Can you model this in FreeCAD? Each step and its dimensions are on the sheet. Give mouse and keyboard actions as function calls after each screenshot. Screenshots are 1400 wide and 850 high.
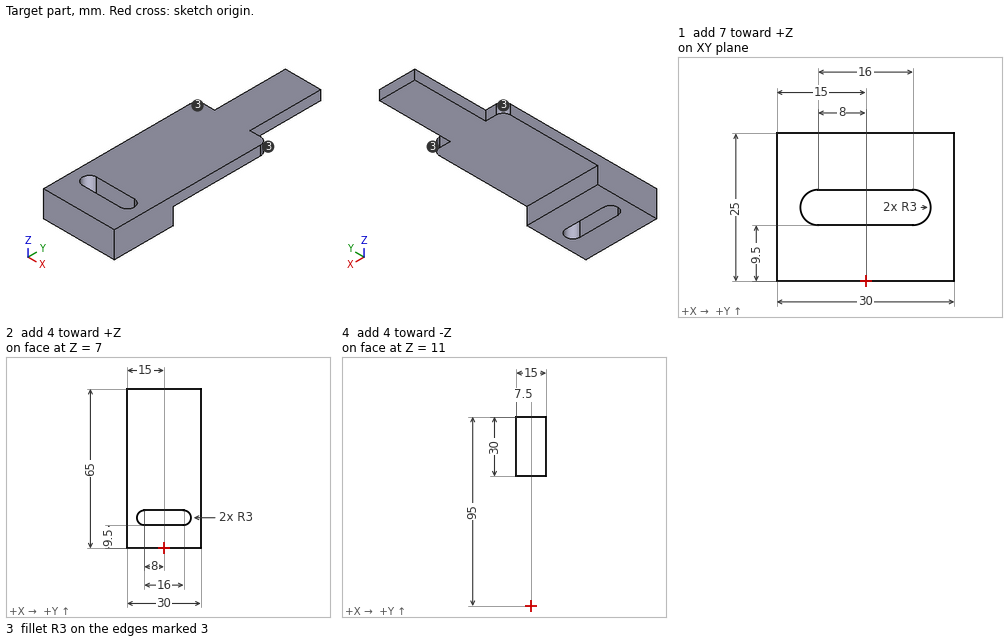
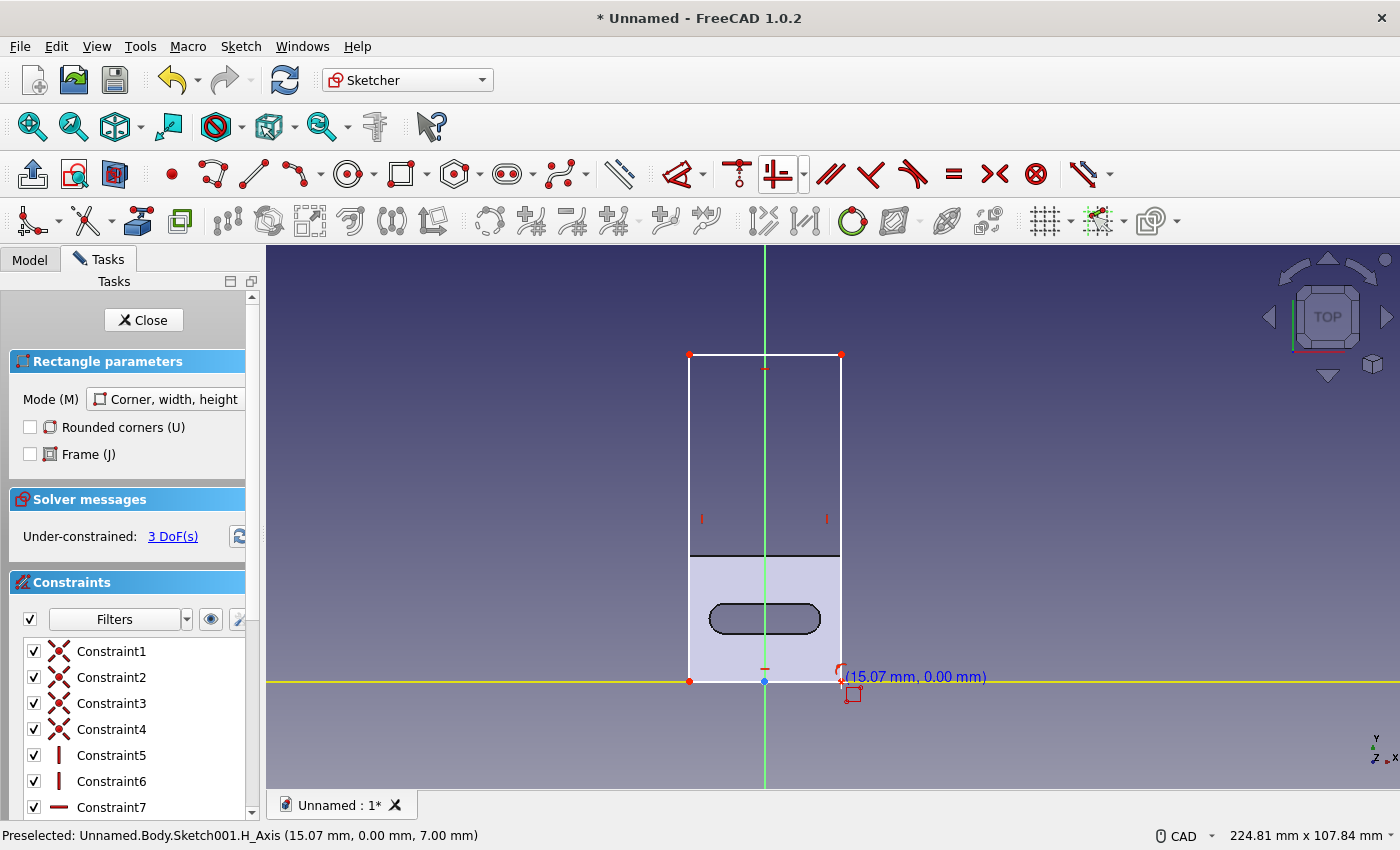
click(506, 174)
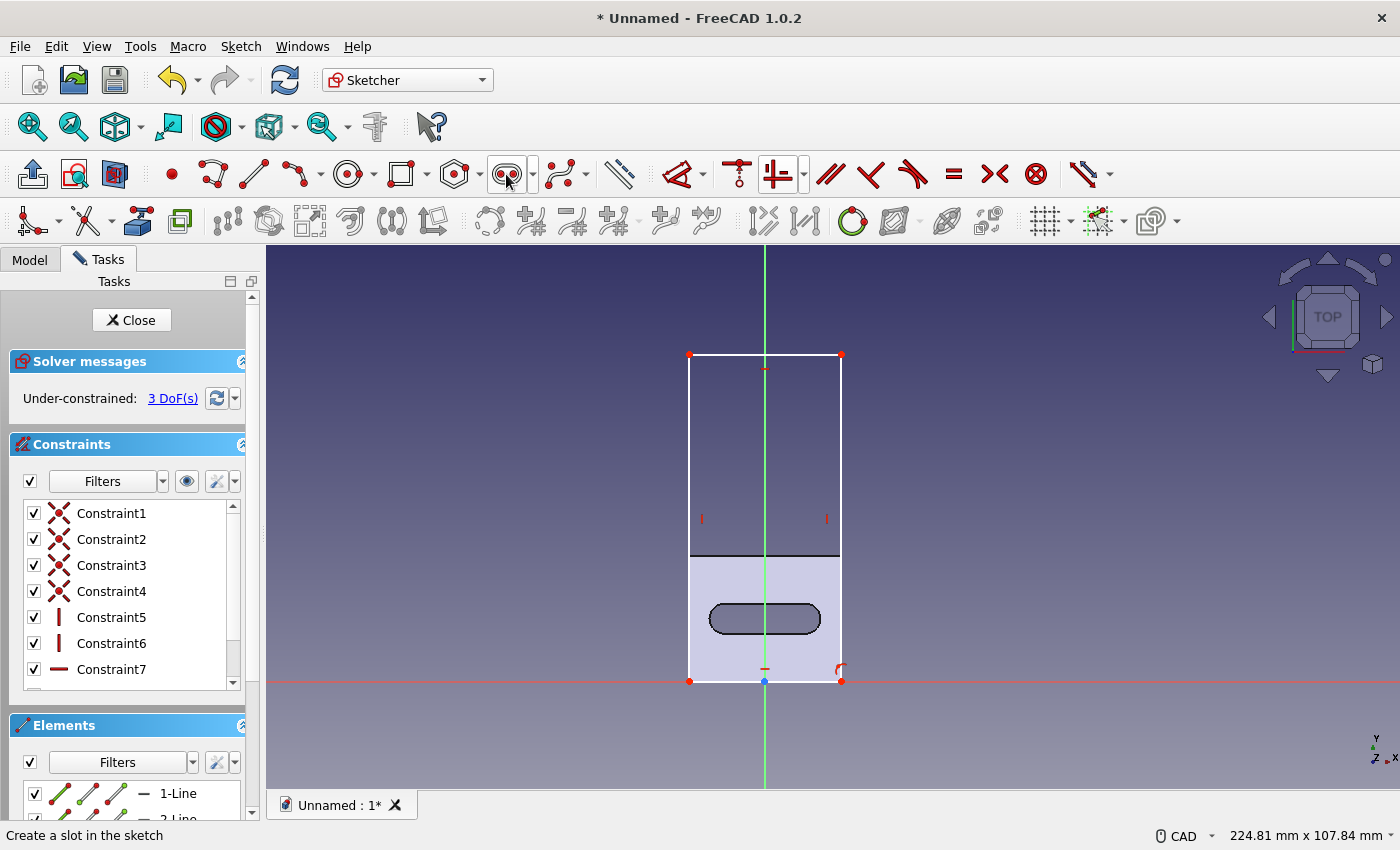
scroll(725, 619, up, 3)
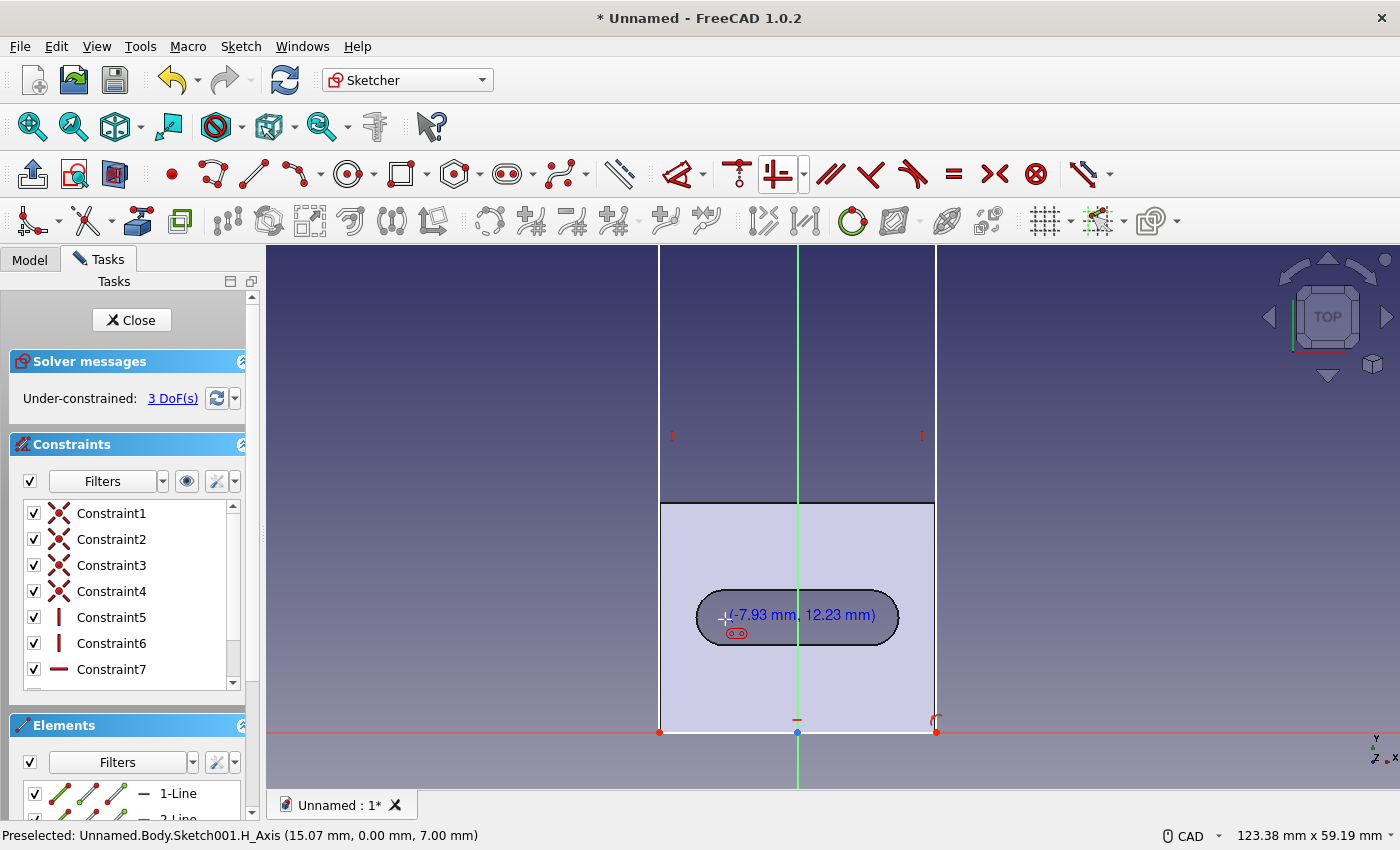
click(724, 618)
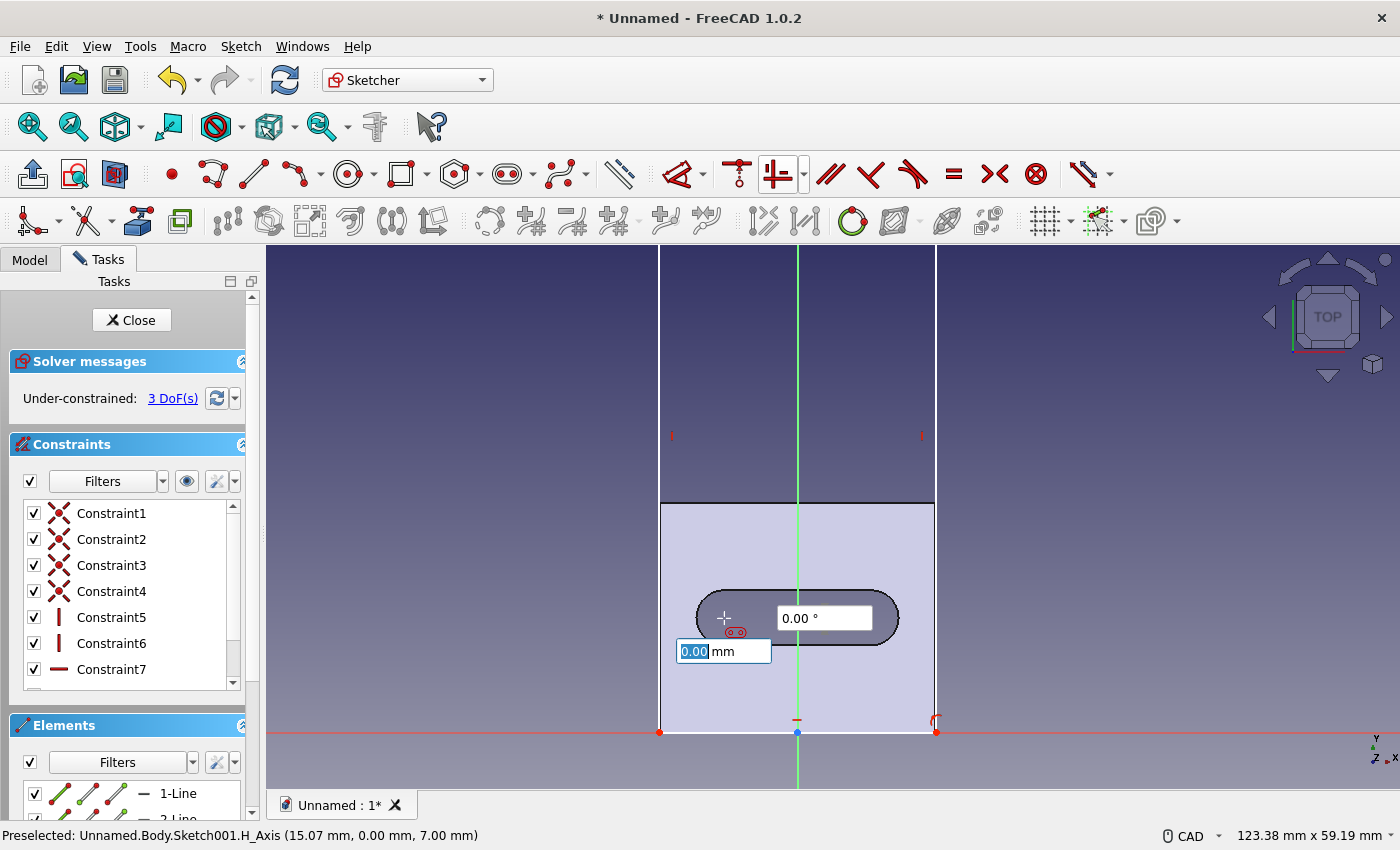
click(871, 618)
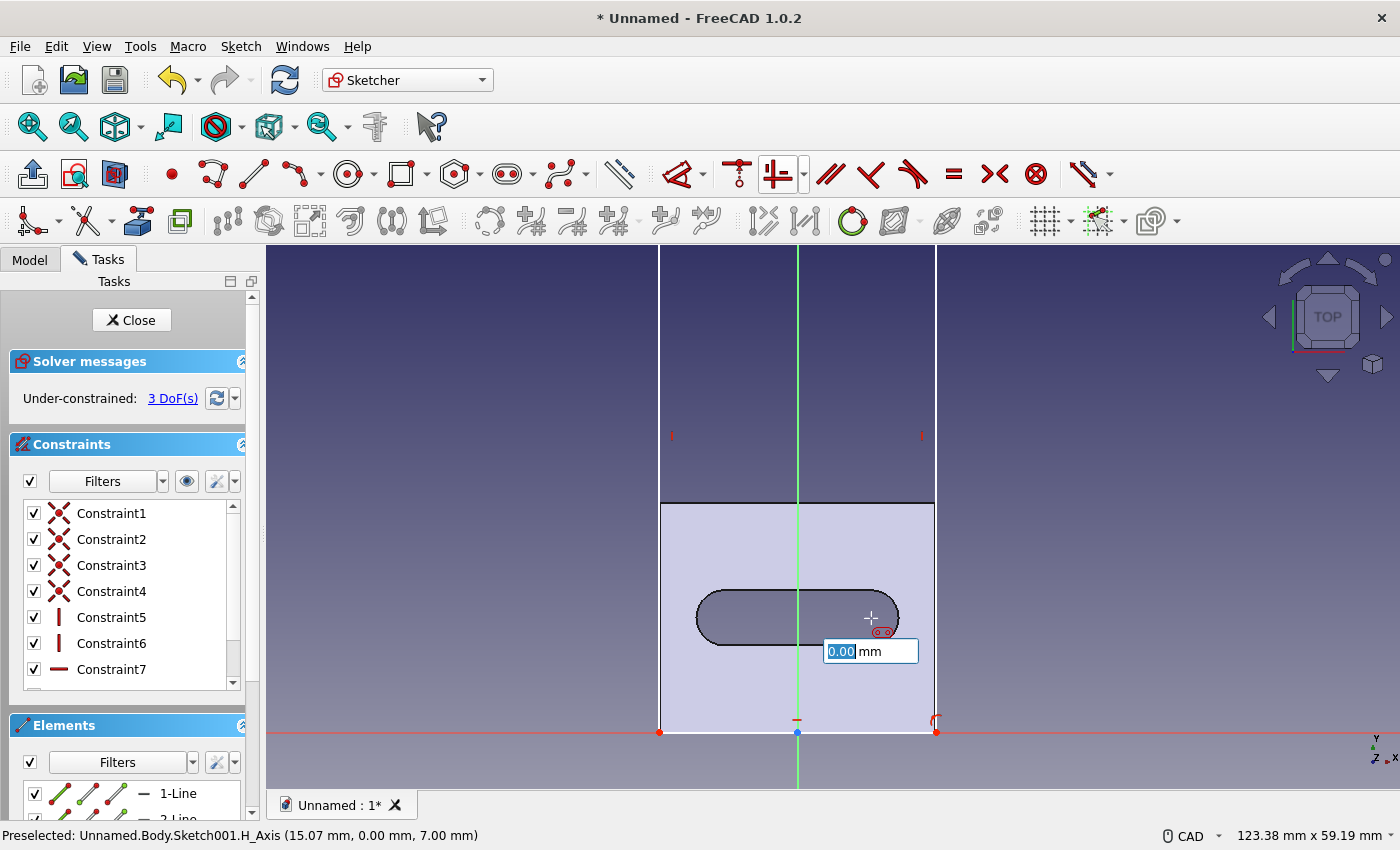
click(820, 645)
key(Escape)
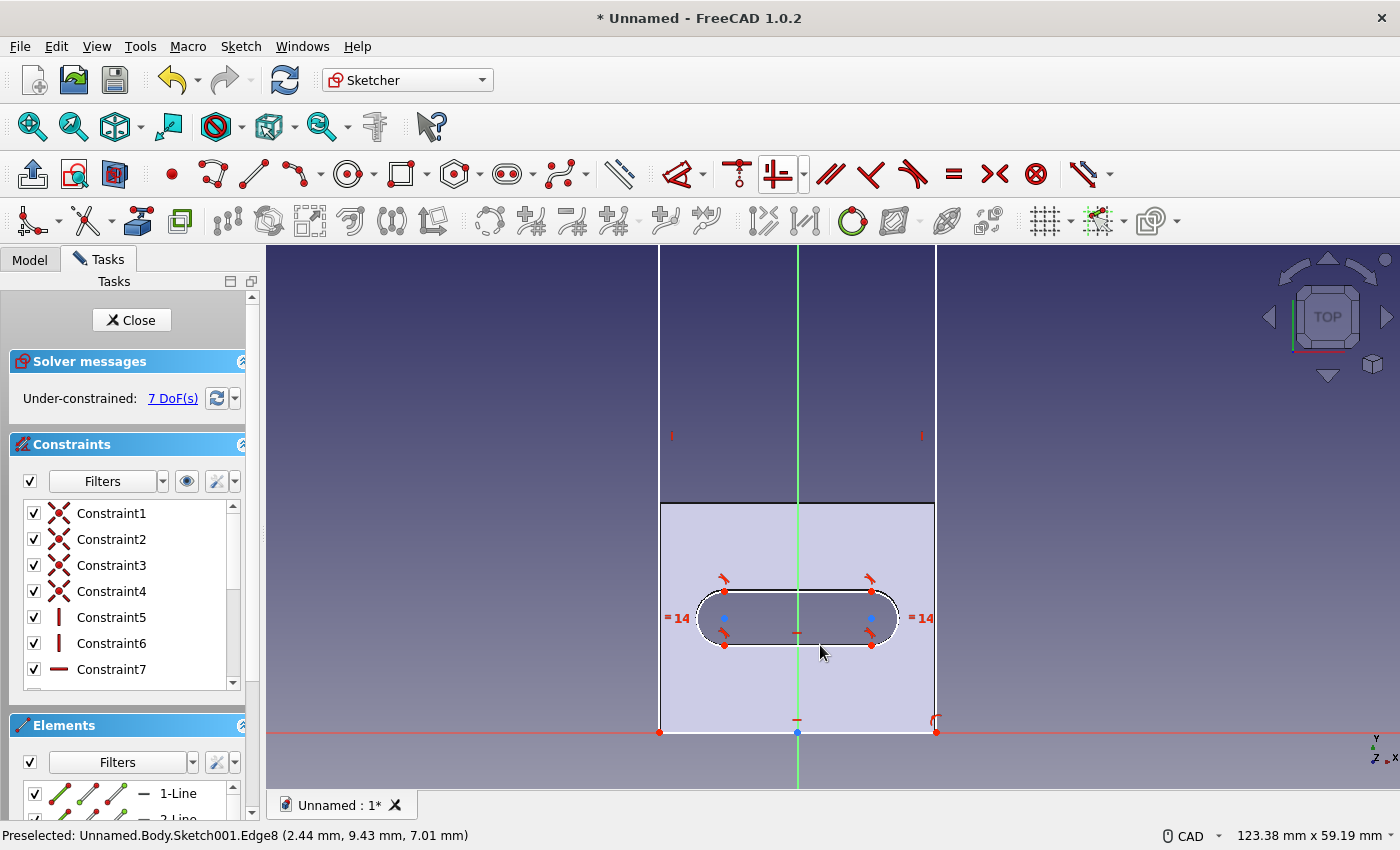
click(676, 174)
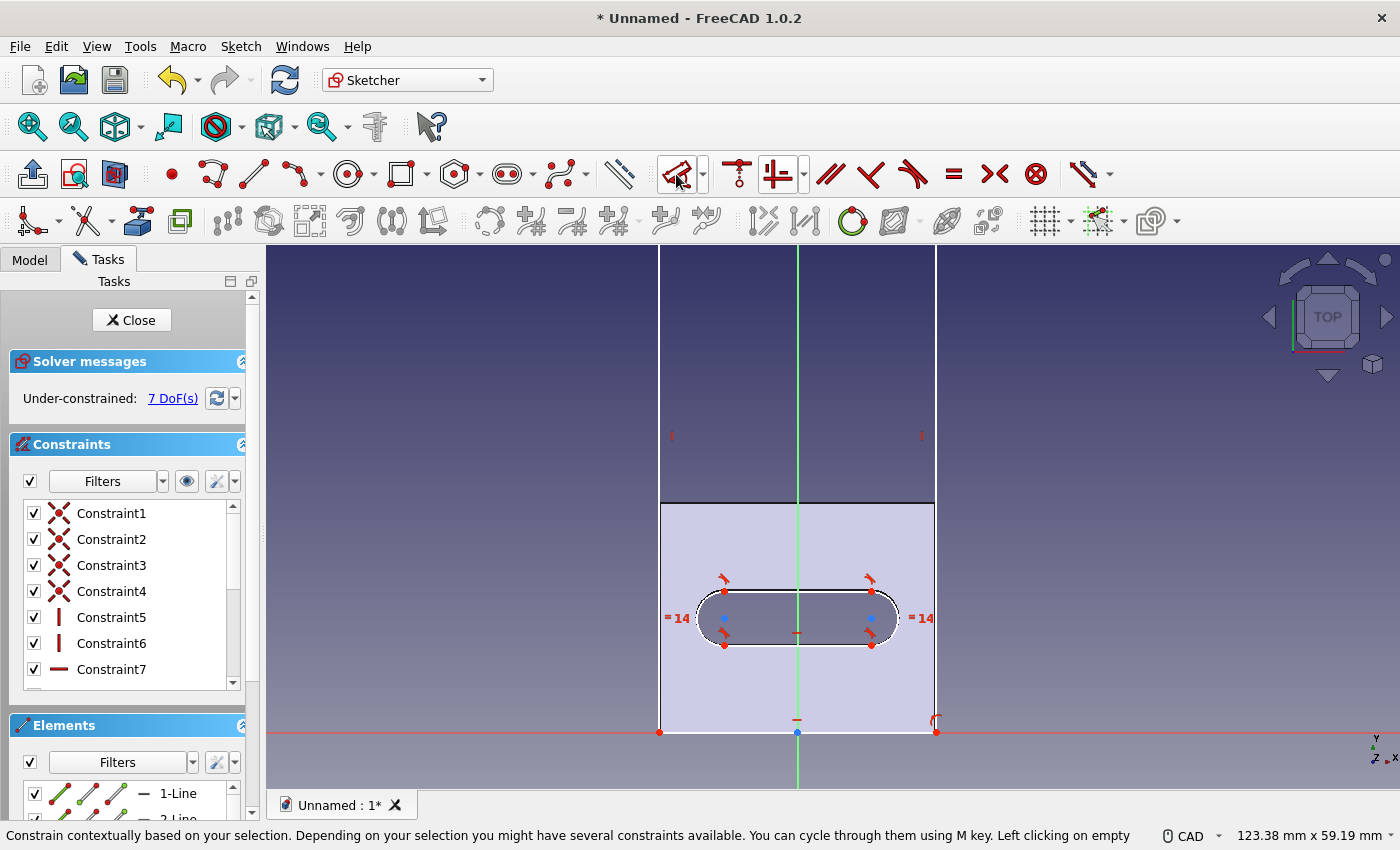
scroll(702, 603, up, 2)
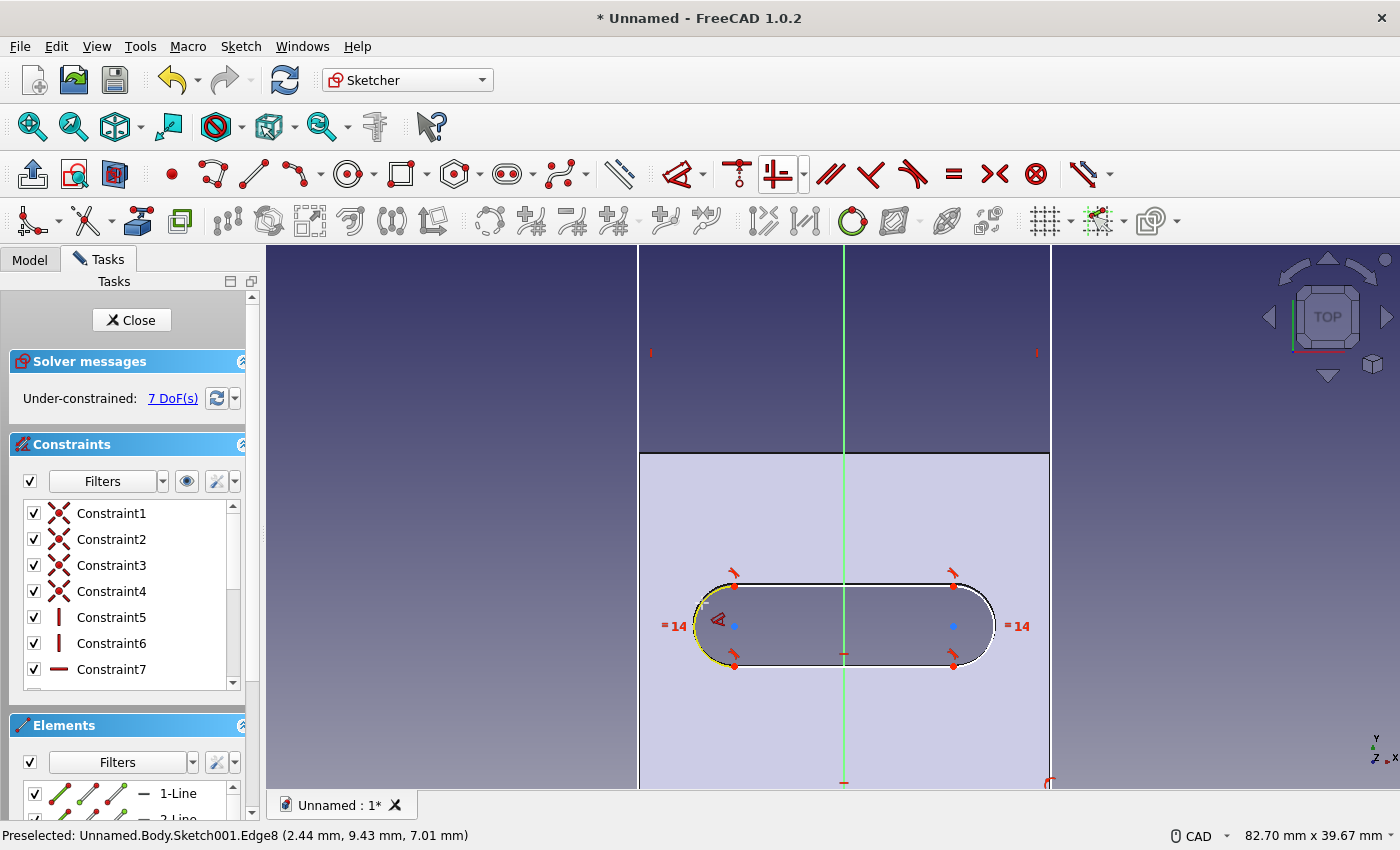
click(702, 603)
click(676, 584)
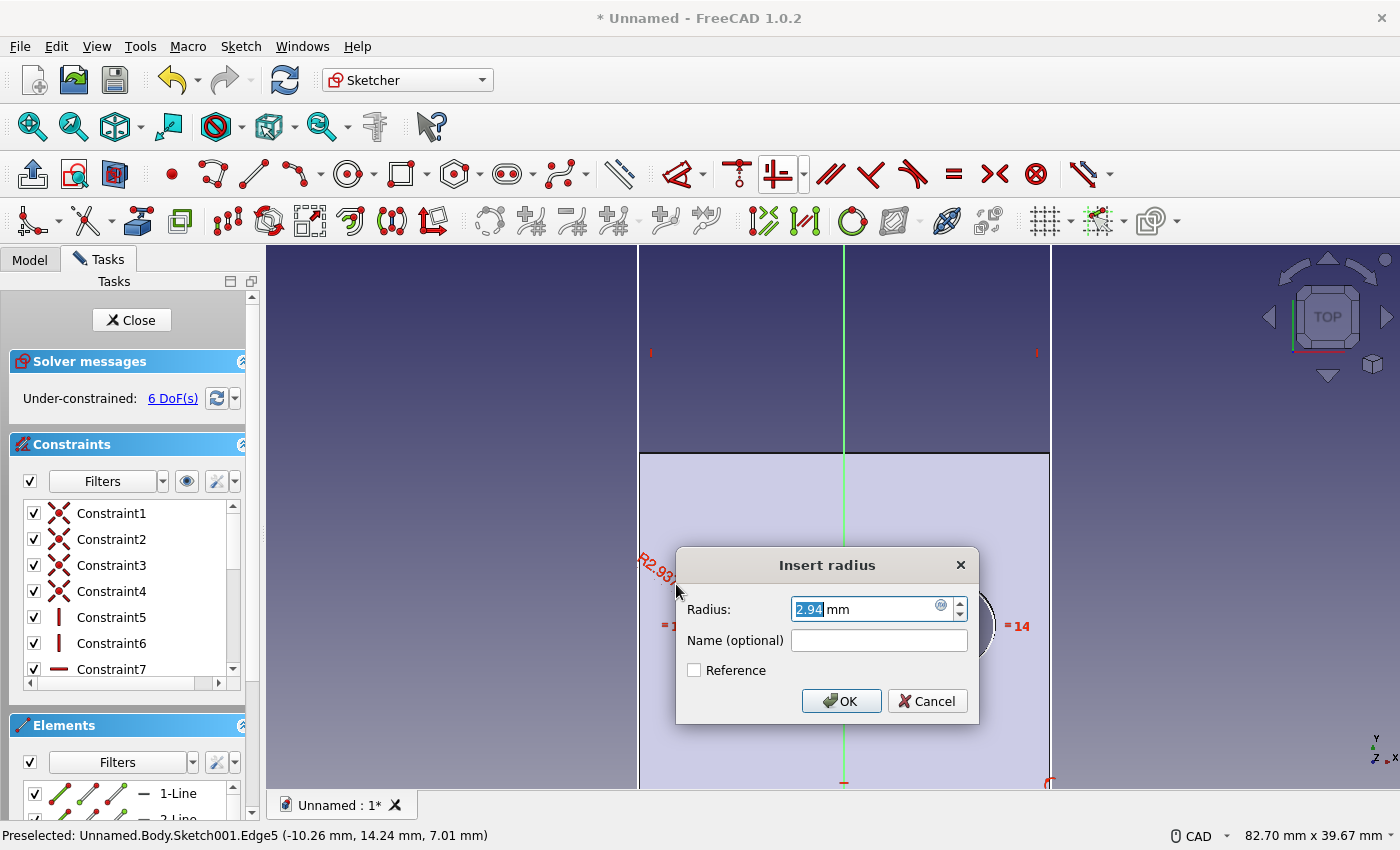
text(3)
key(Return)